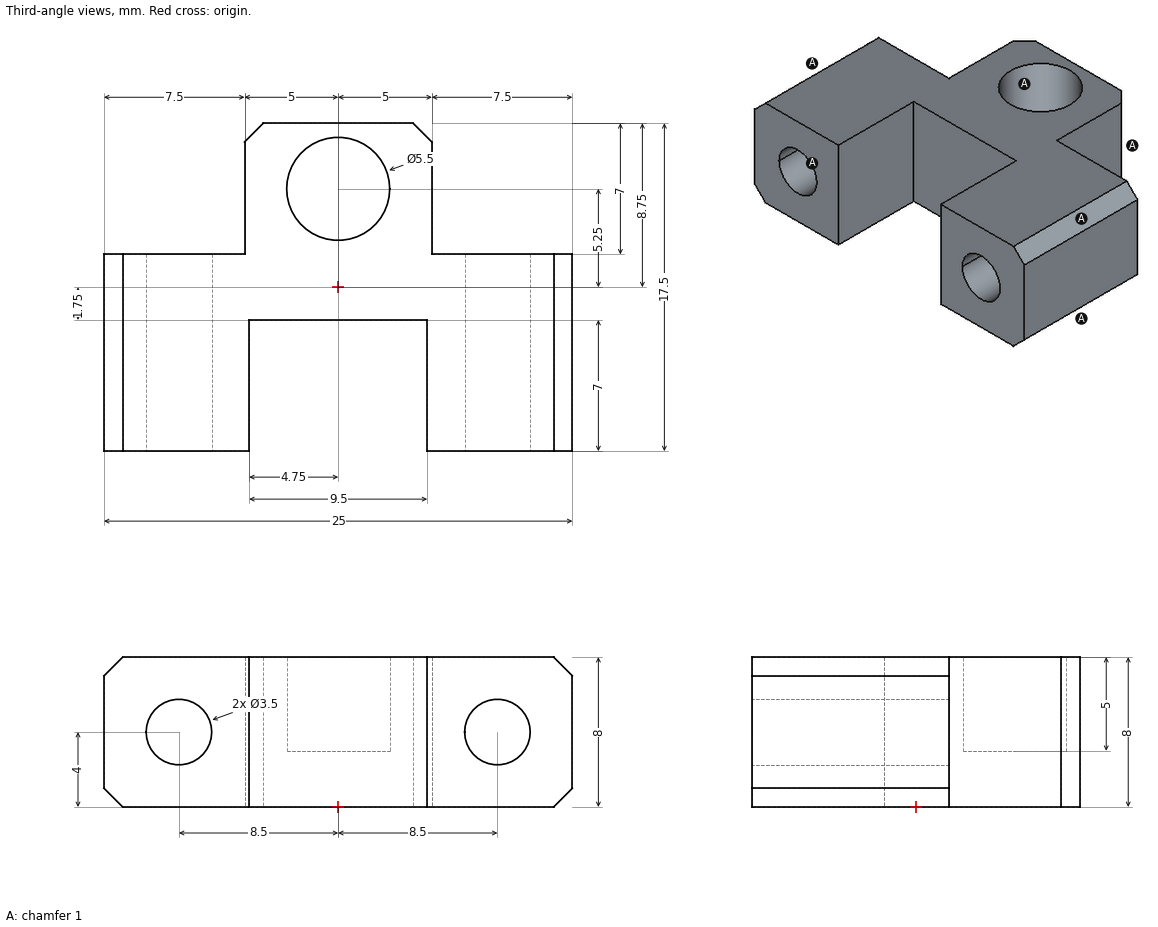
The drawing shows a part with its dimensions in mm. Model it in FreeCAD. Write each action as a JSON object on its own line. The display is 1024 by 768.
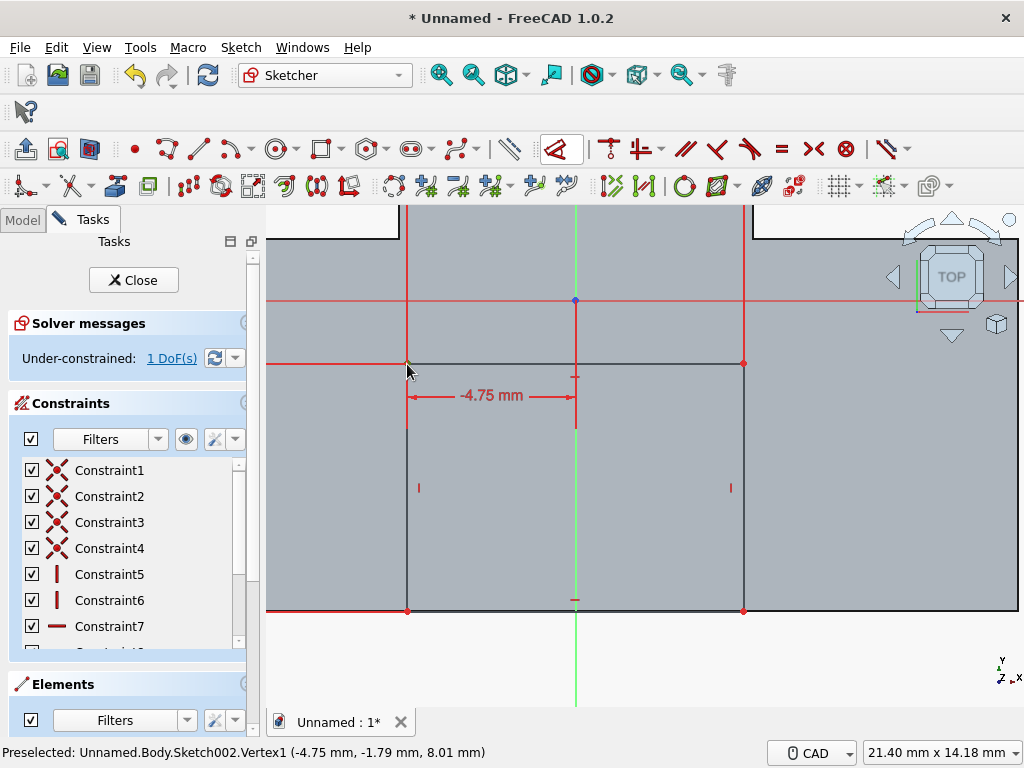
{"action": "key", "text": "i"}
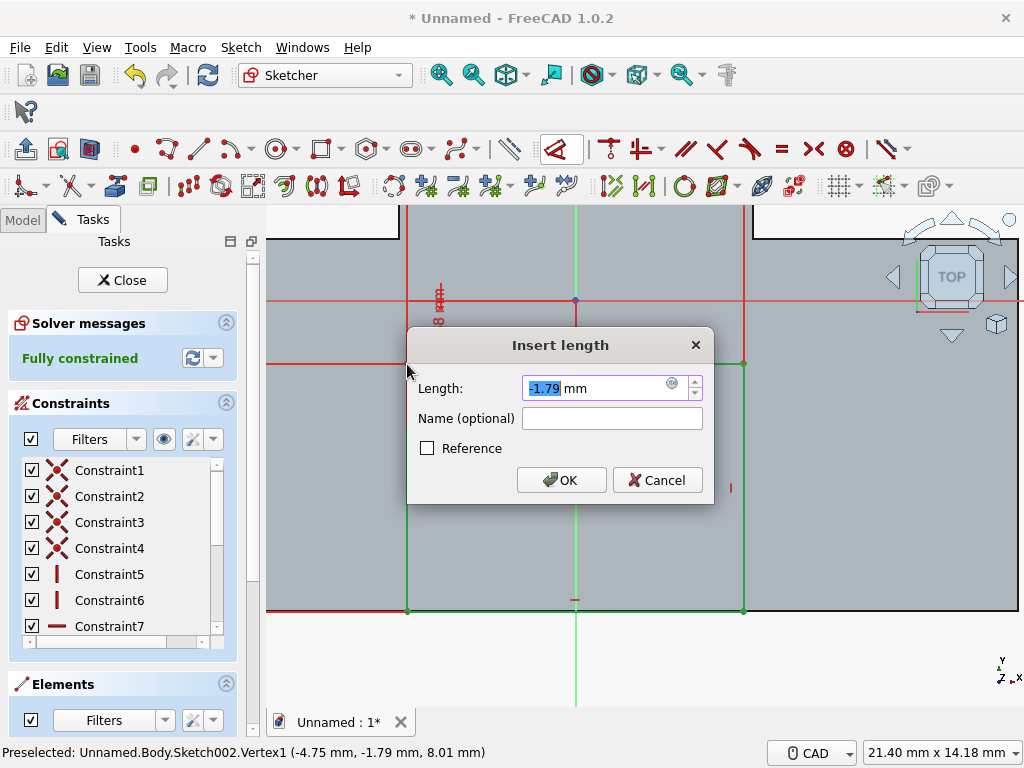
{"action": "type", "text": "-1.75"}
{"action": "key", "text": "Return"}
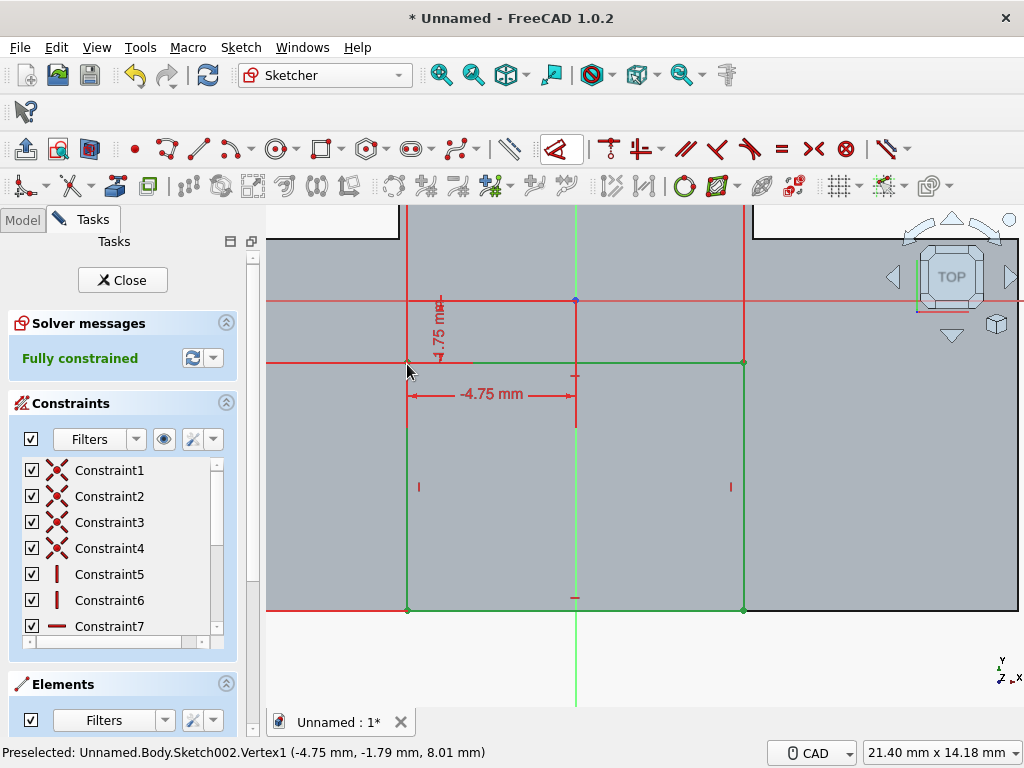
{"action": "left_click", "coordinate": [123, 280]}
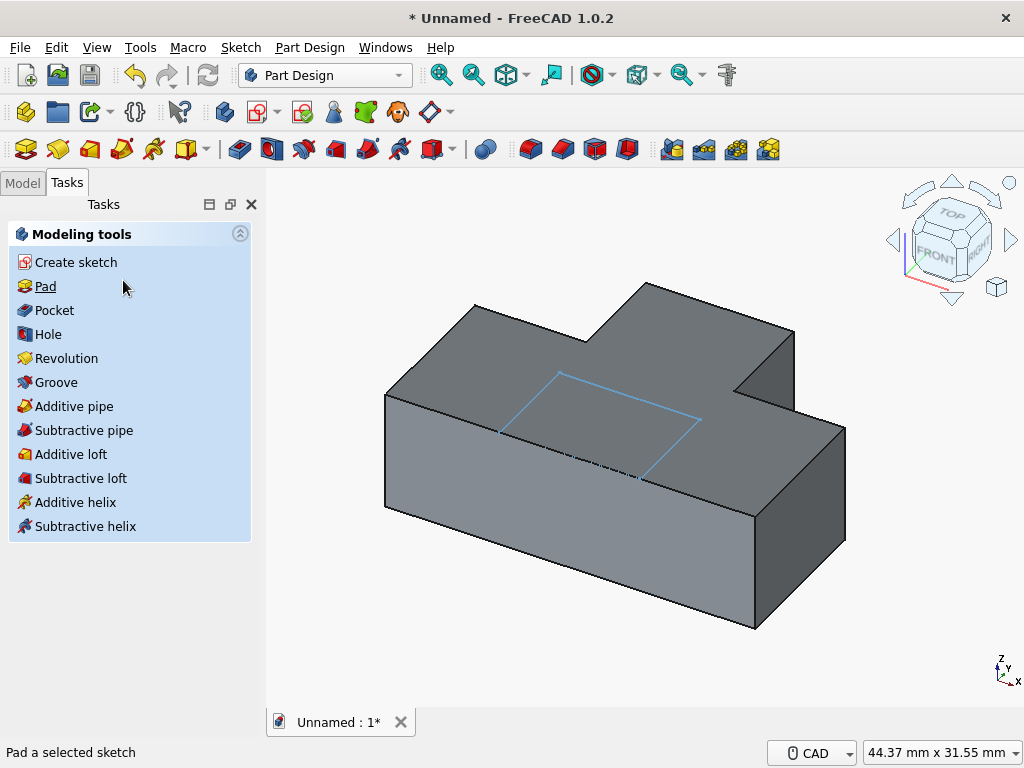
{"action": "left_click", "coordinate": [240, 150]}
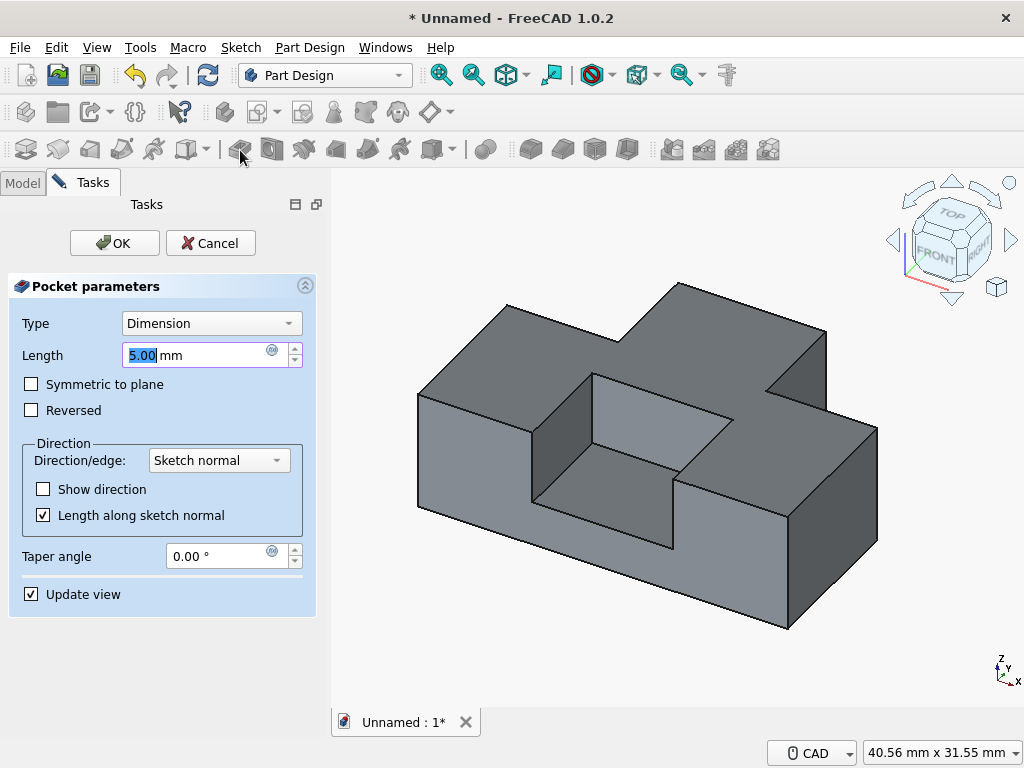
{"action": "left_click", "coordinate": [212, 324]}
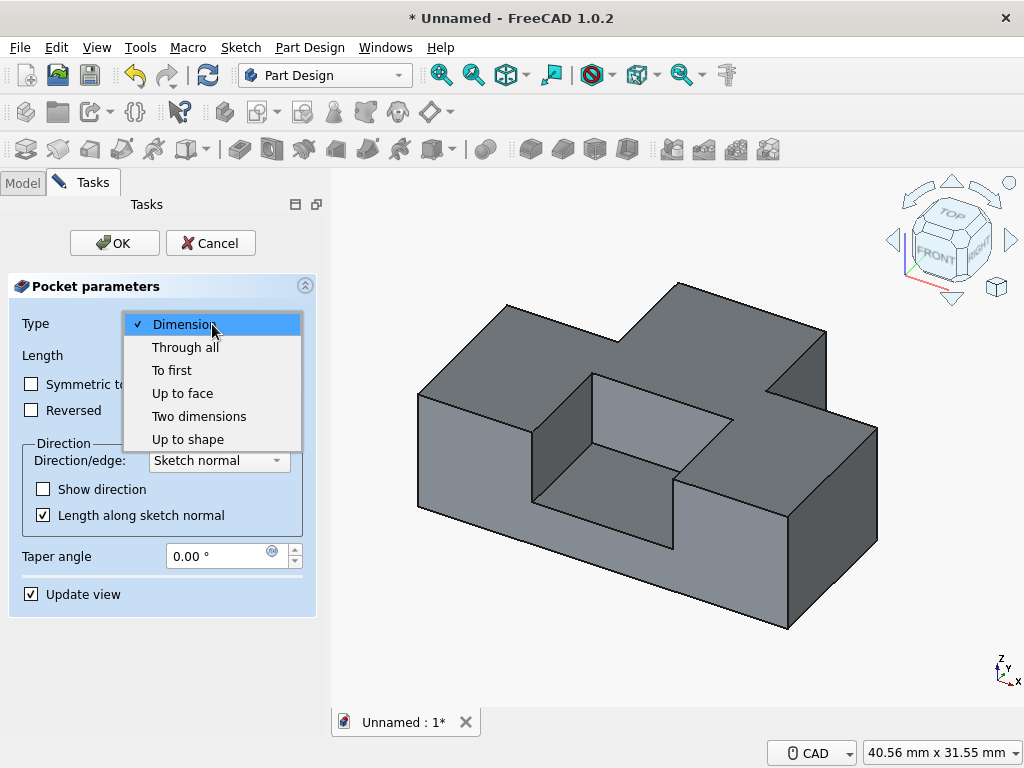
{"action": "left_click", "coordinate": [212, 348]}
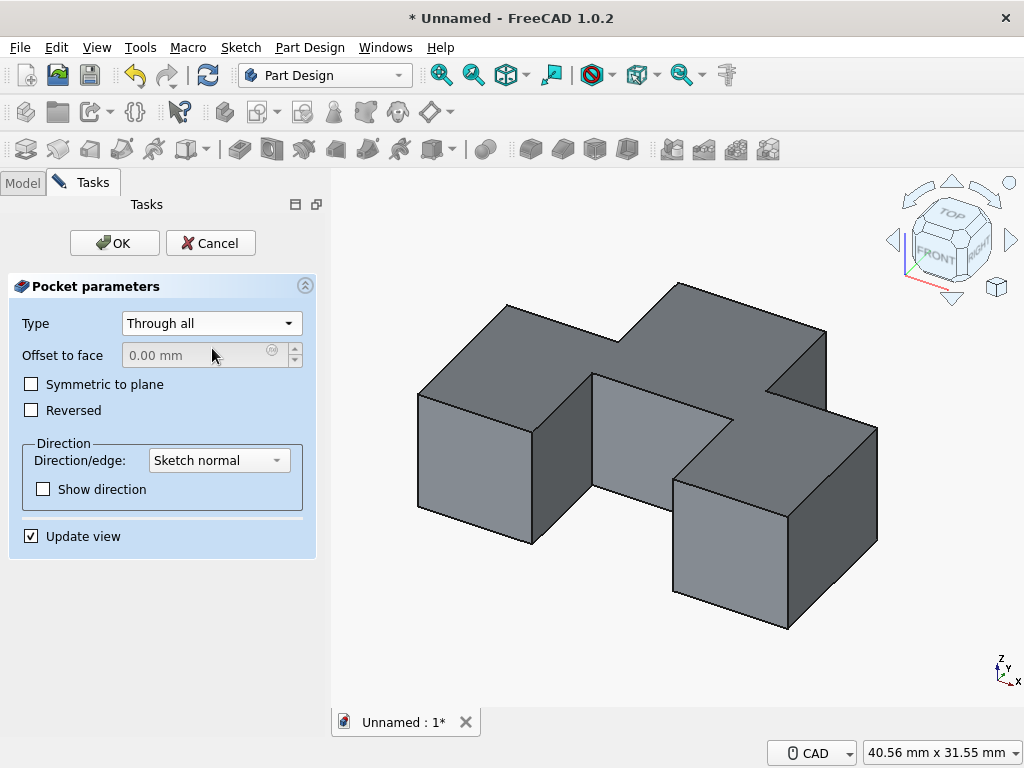
{"action": "left_click", "coordinate": [115, 243]}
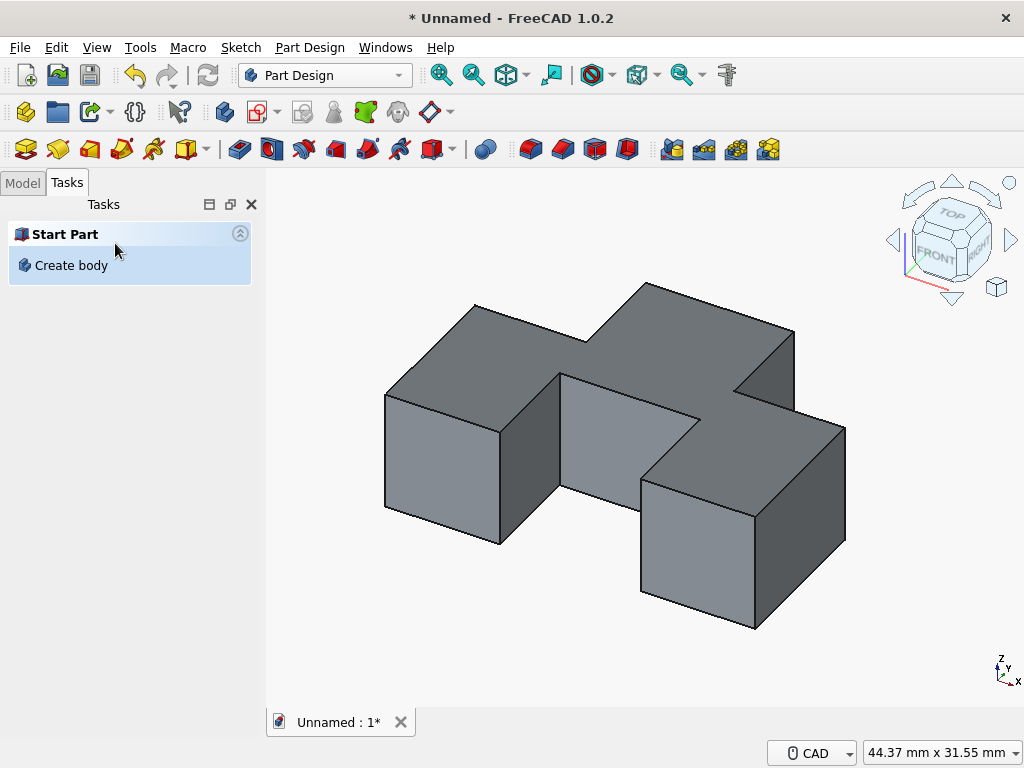
{"action": "left_click", "coordinate": [666, 359]}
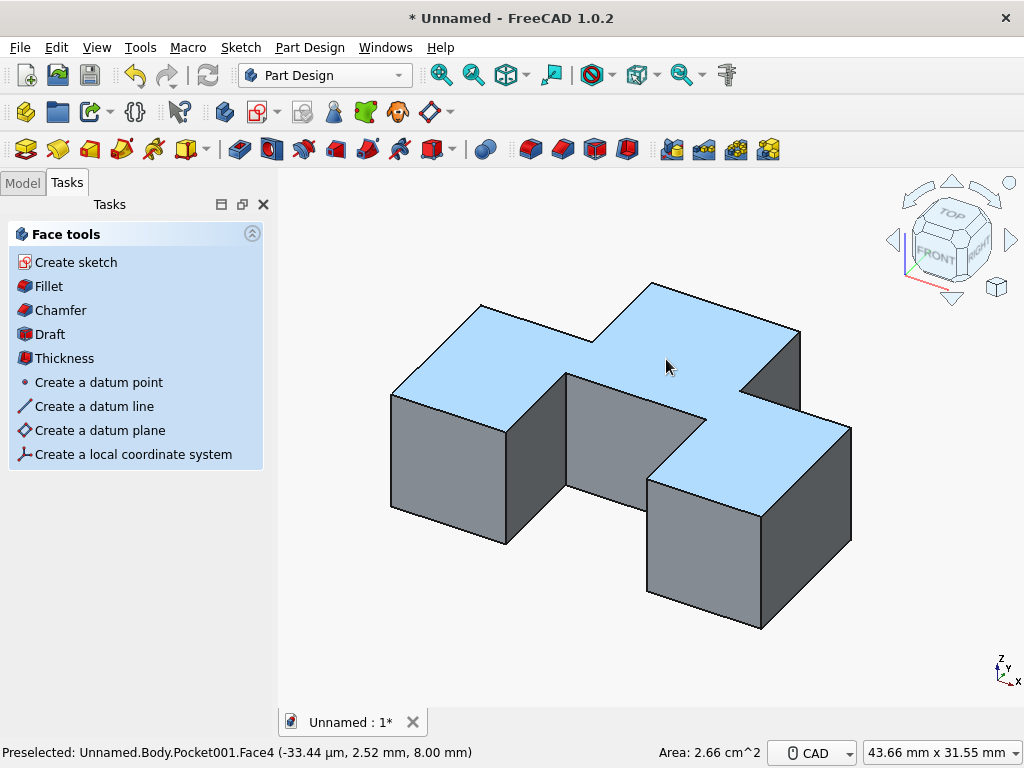
{"action": "left_click", "coordinate": [258, 112]}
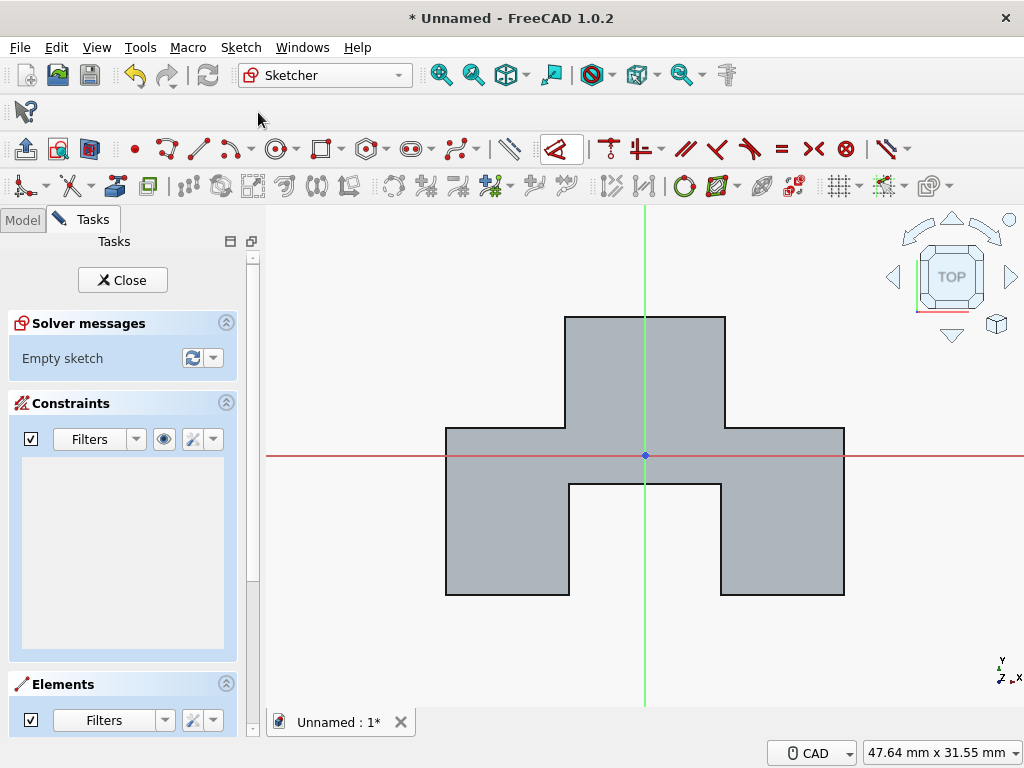
{"action": "scroll", "coordinate": [685, 355], "scroll_direction": "up", "scroll_amount": 5}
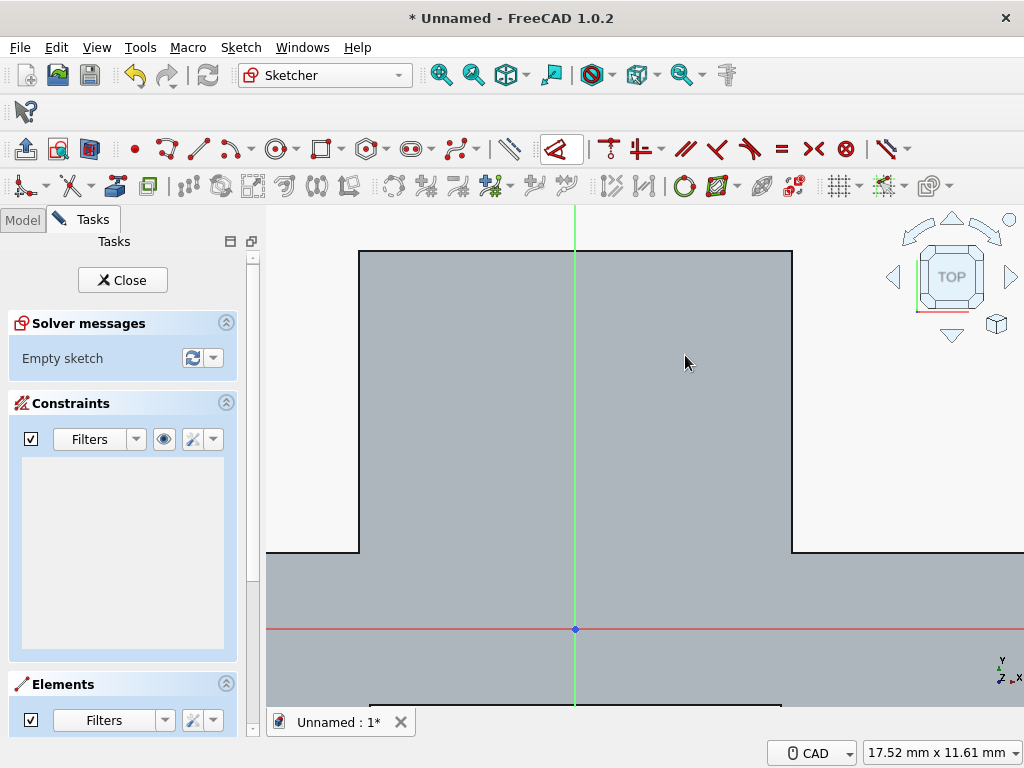
{"action": "key", "text": "g c"}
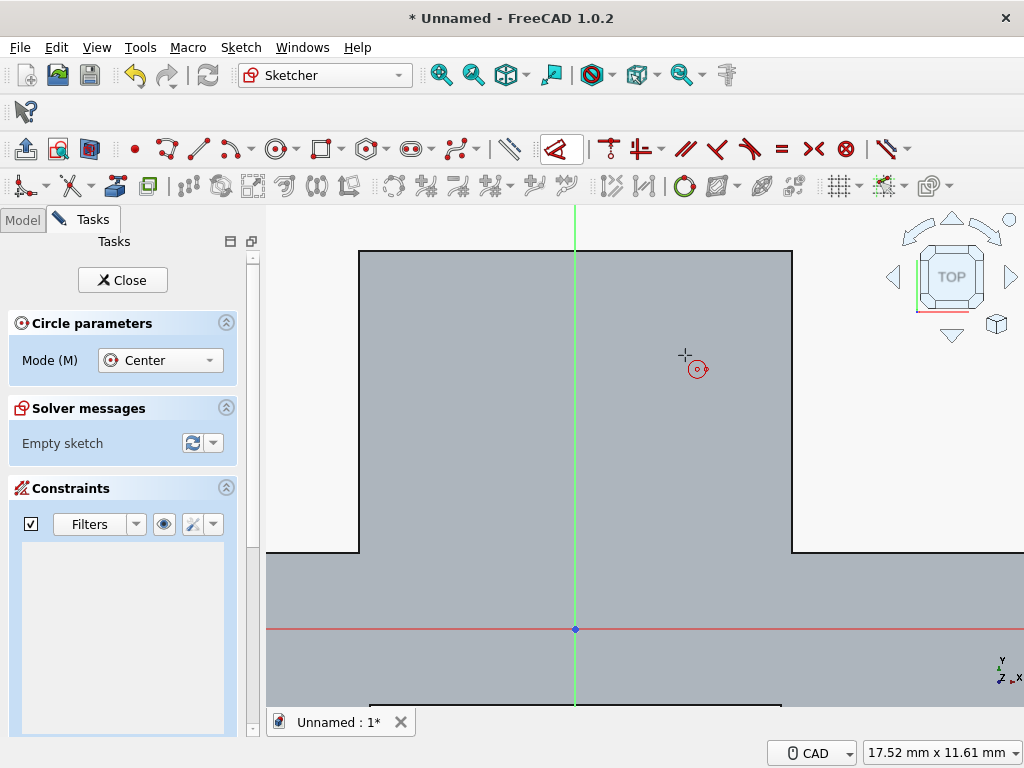
{"action": "left_click", "coordinate": [575, 402]}
{"action": "mouse_move", "coordinate": [659, 318]}